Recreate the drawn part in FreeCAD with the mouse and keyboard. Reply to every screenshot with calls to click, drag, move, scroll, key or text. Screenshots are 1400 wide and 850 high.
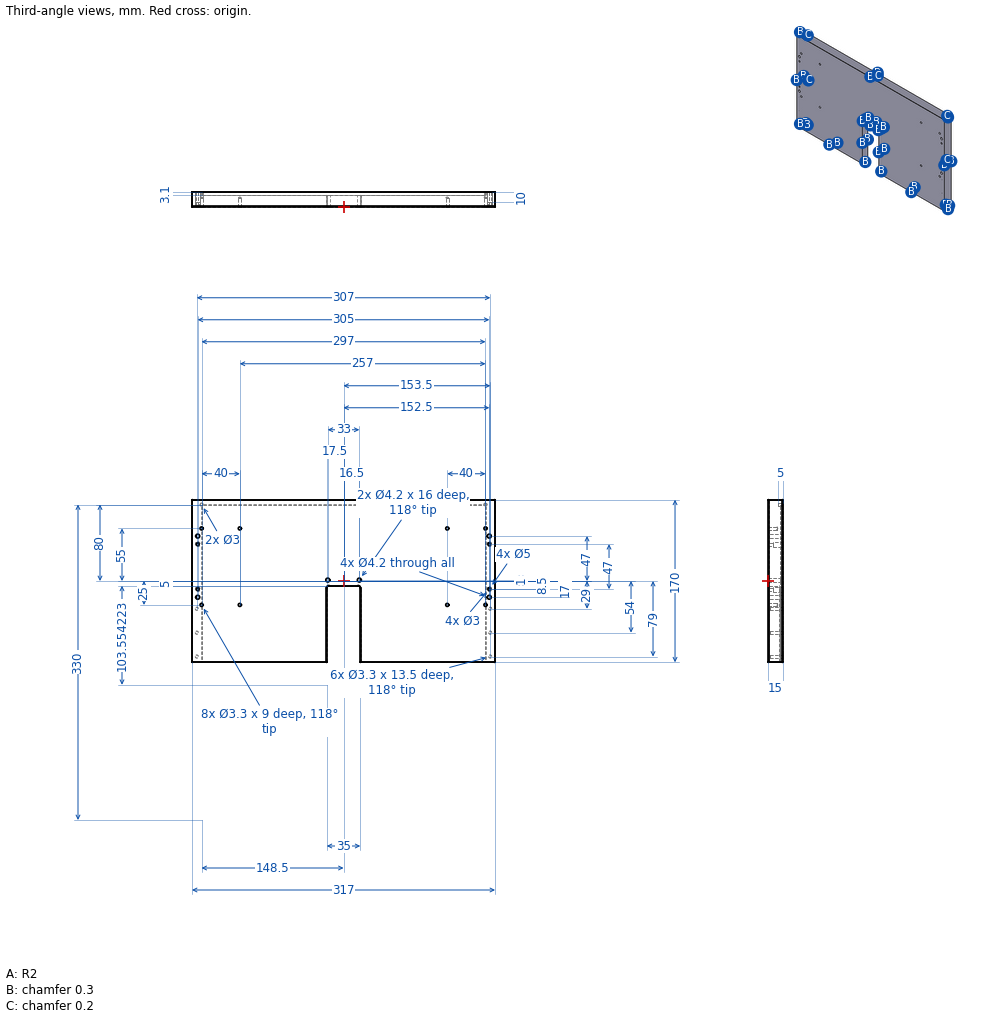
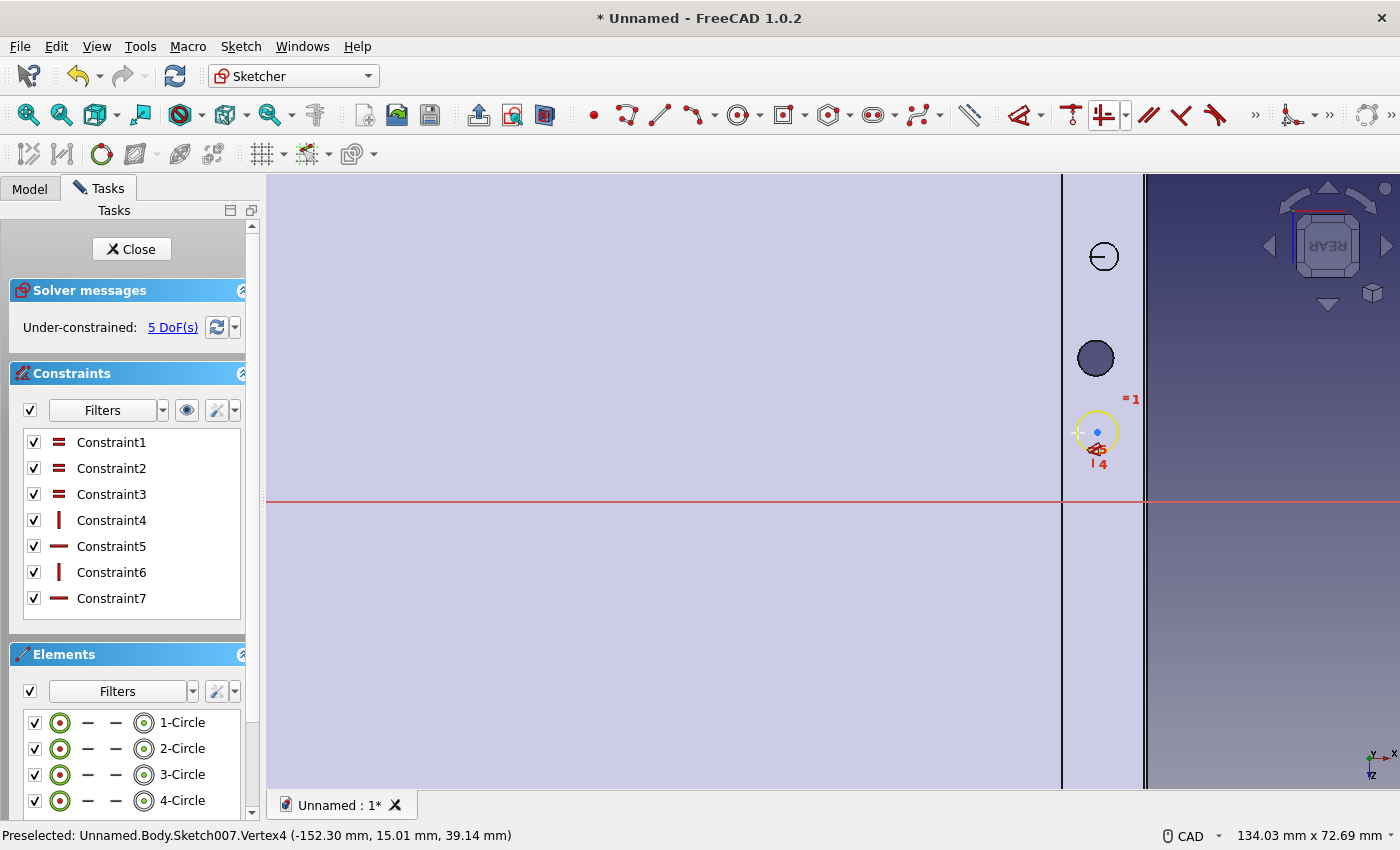
click(1076, 432)
click(1044, 432)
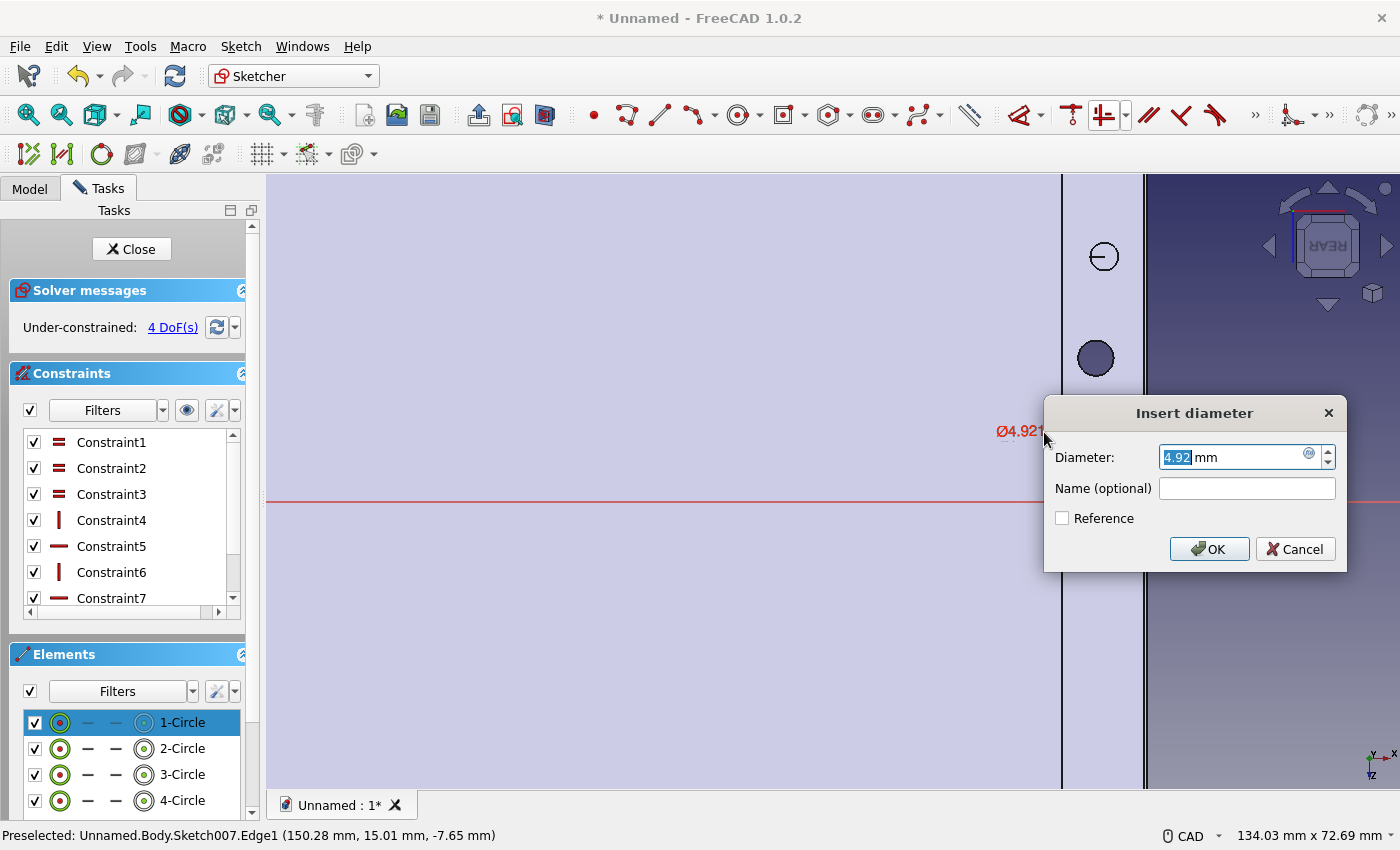
text(5)
key(Return)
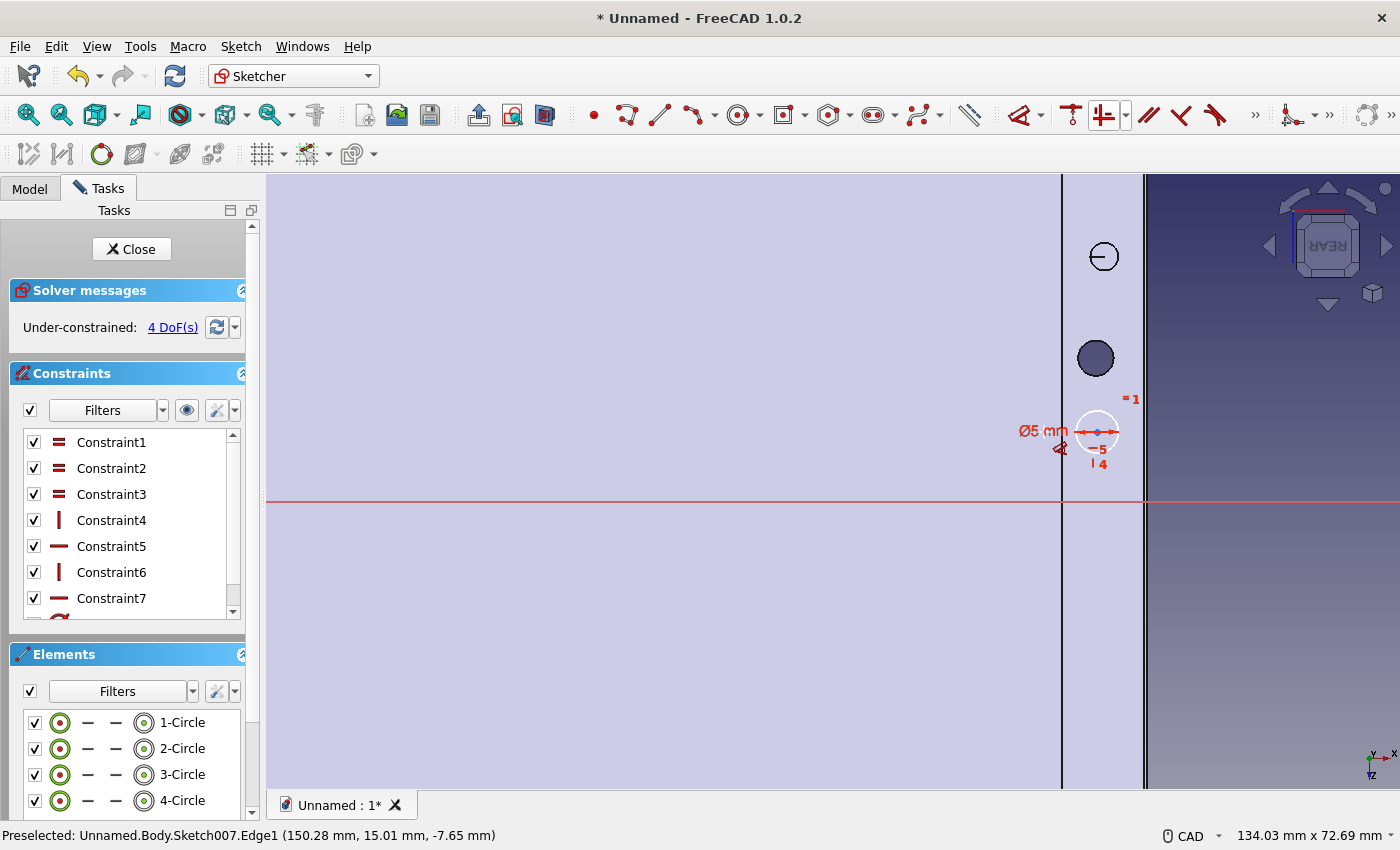
click(1097, 432)
click(1131, 467)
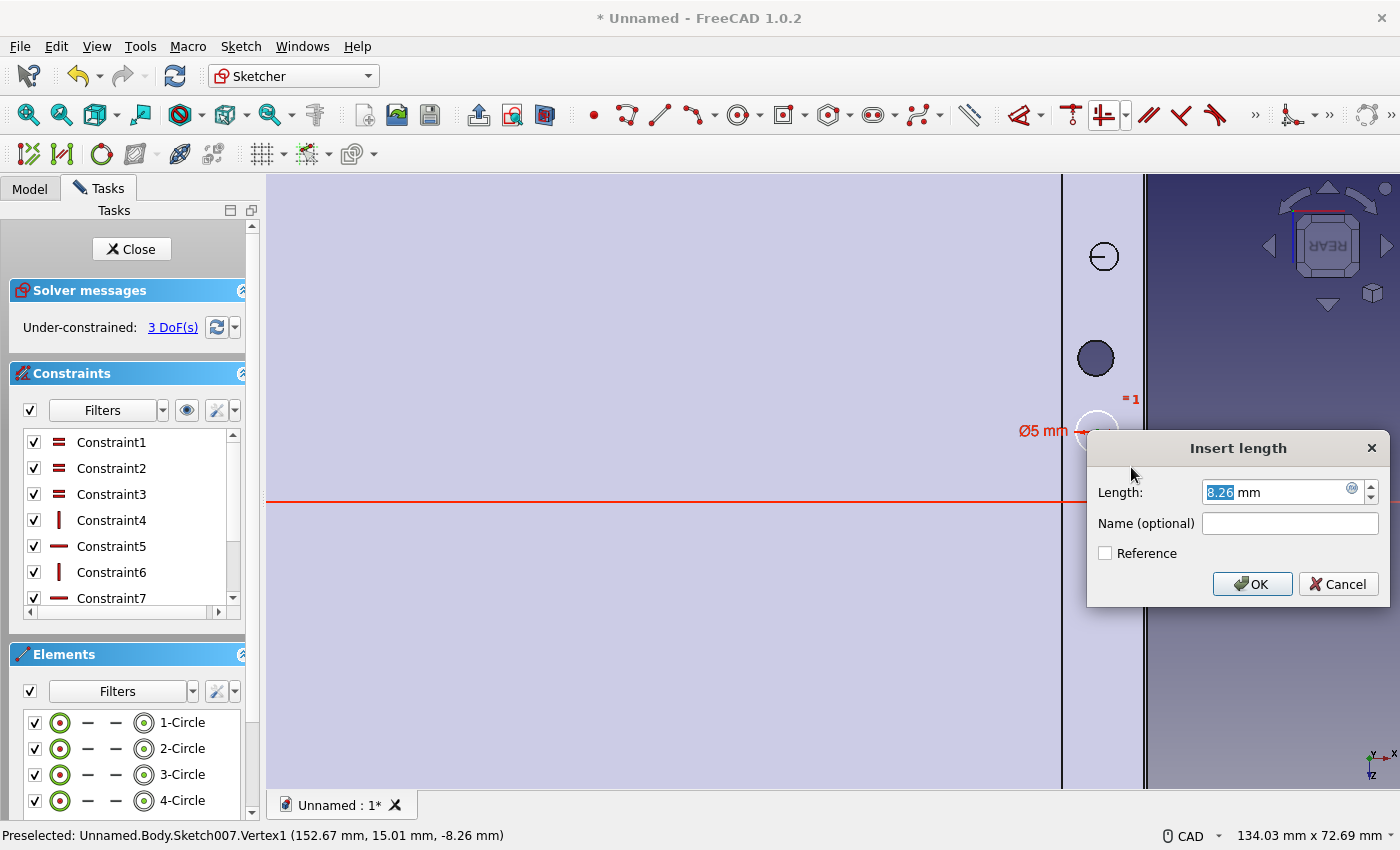
text(8.5)
key(Return)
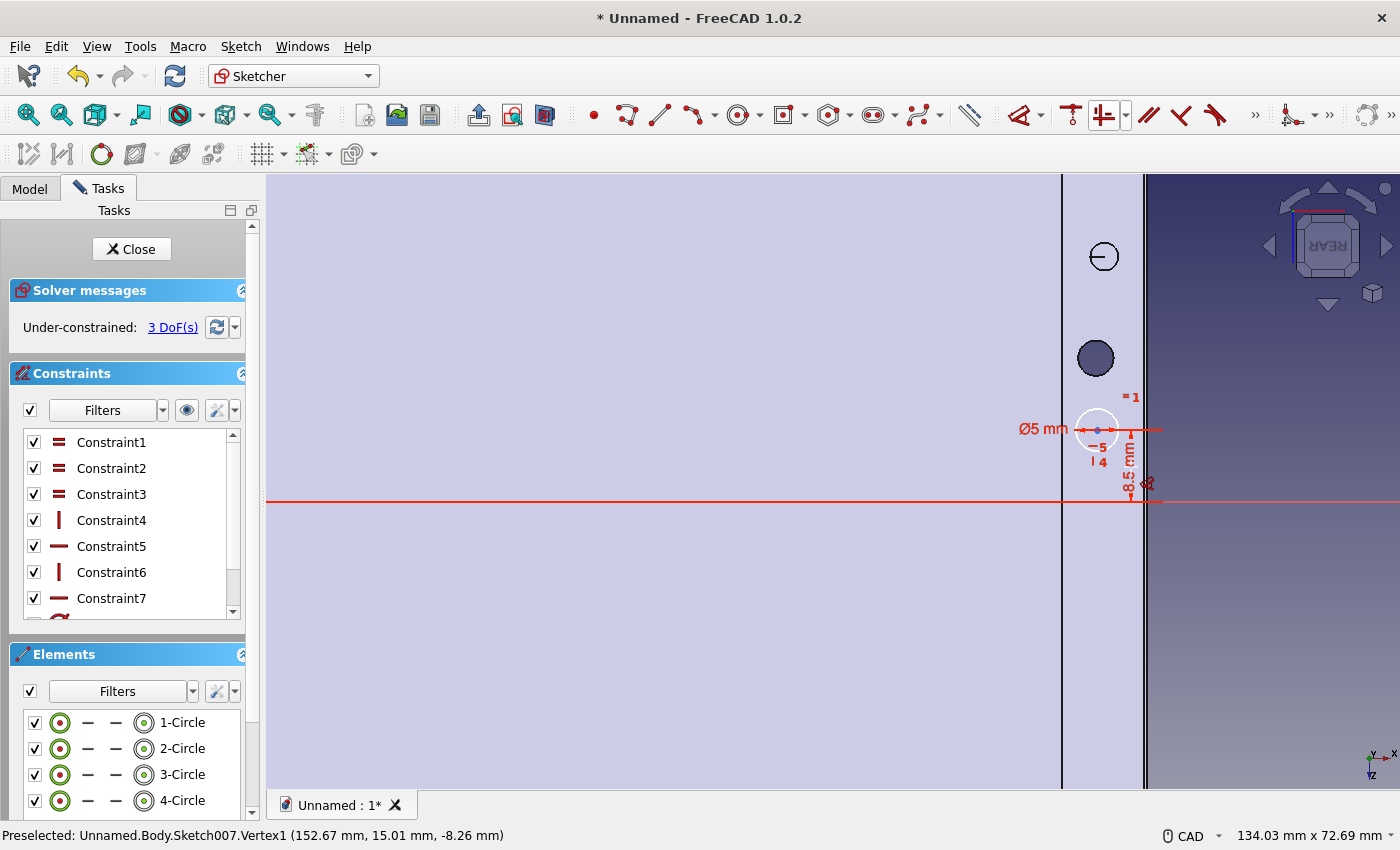
scroll(1078, 433, down, 7)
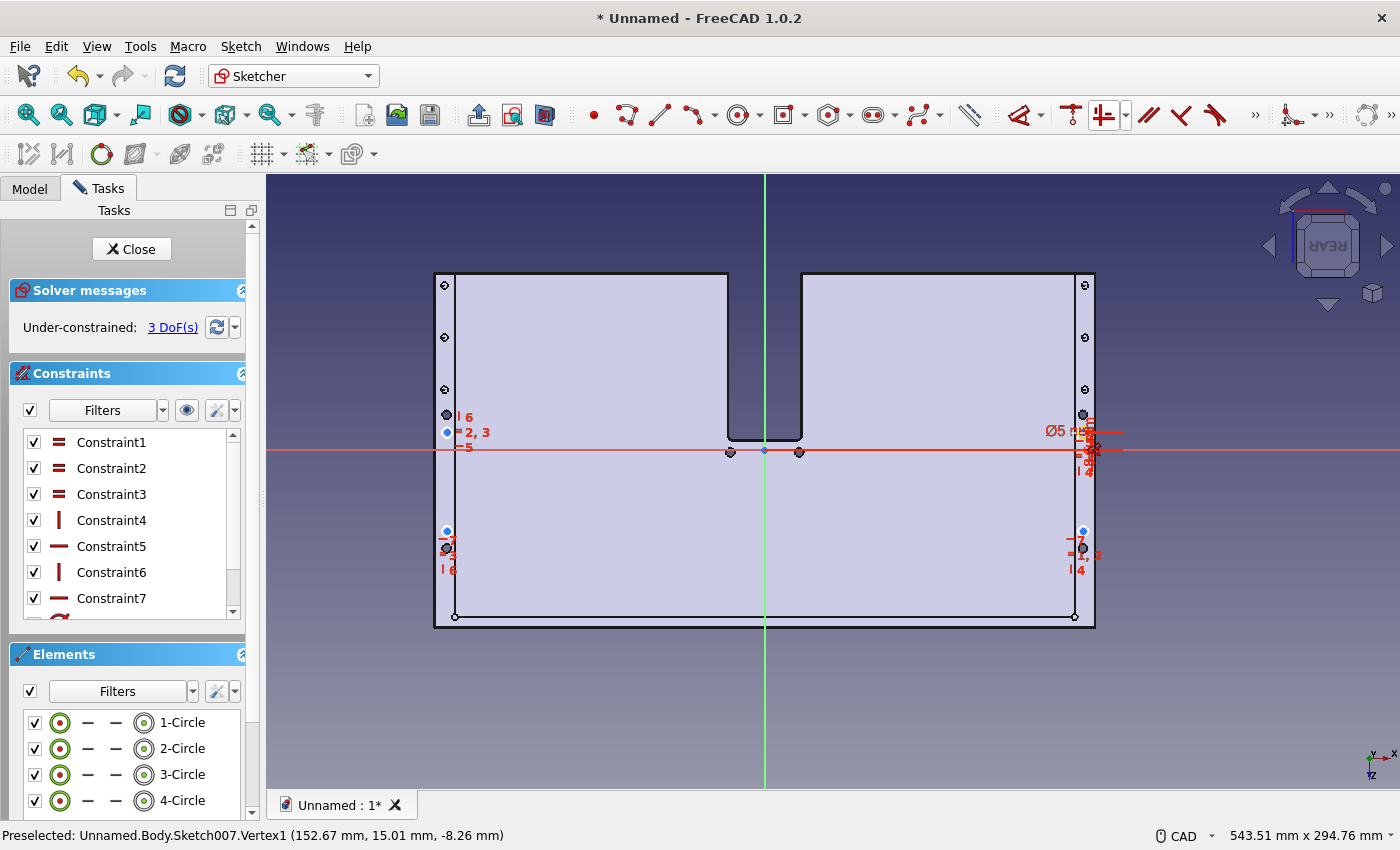
click(1083, 433)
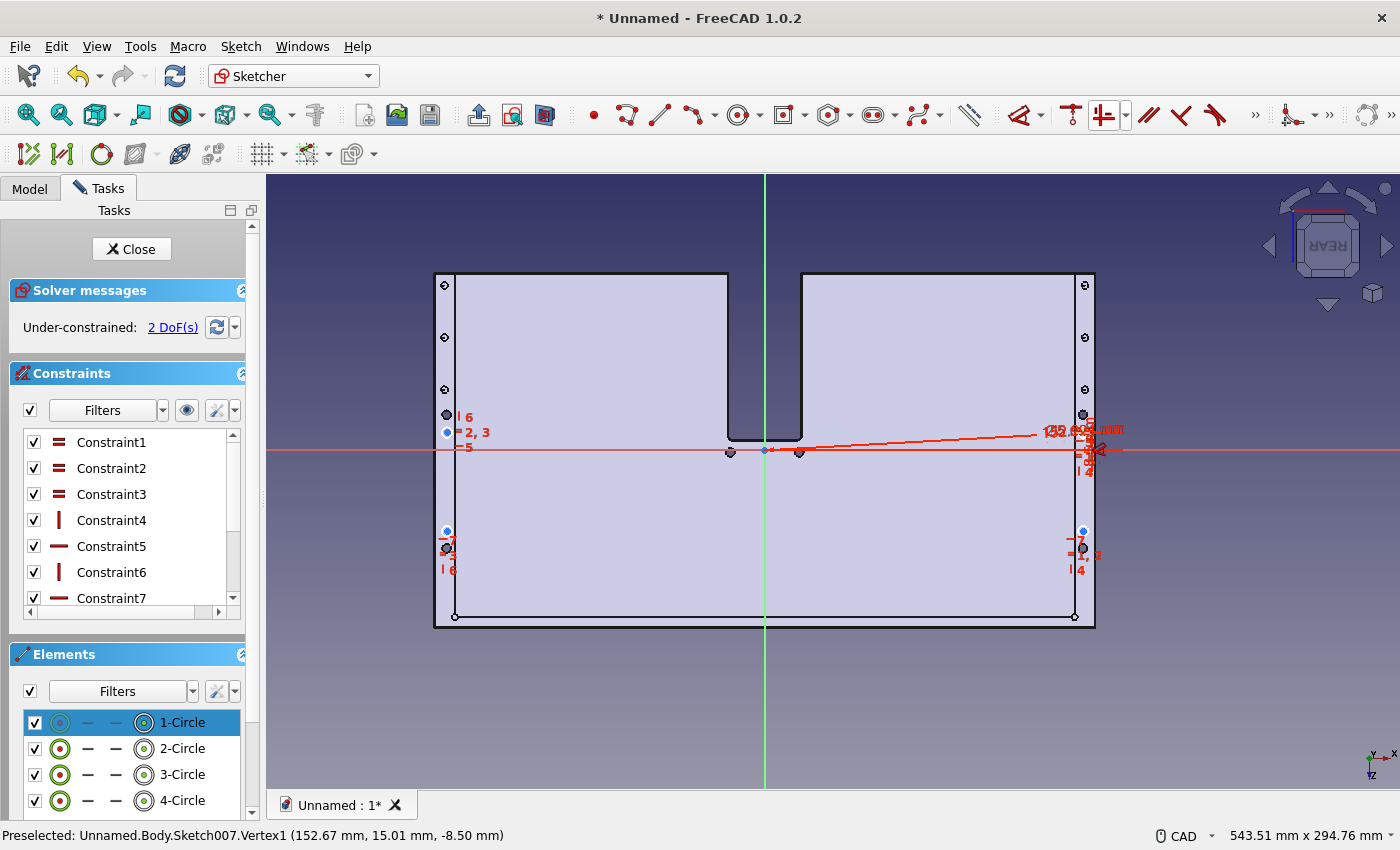
click(1083, 531)
click(1117, 482)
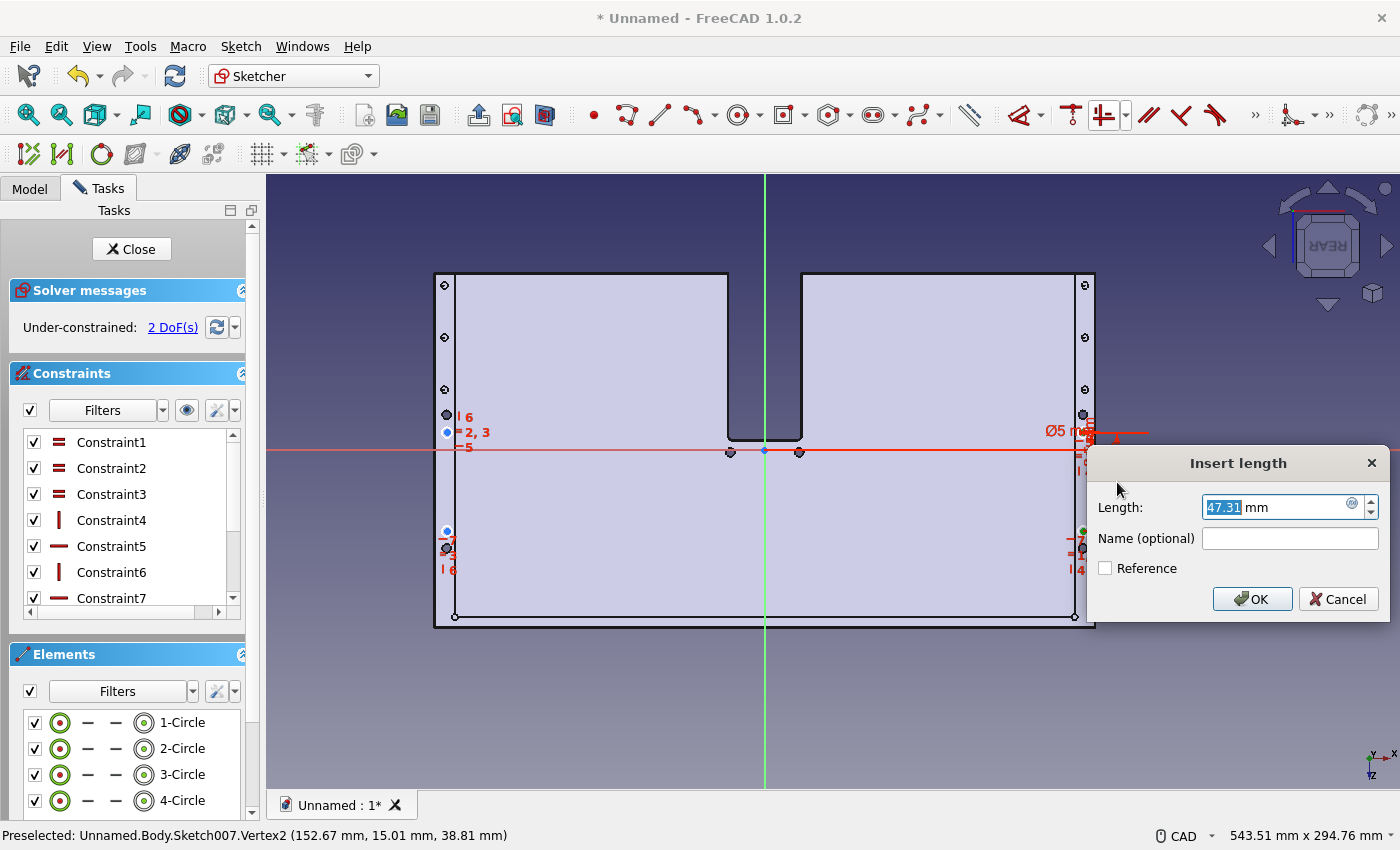
text(47)
key(Return)